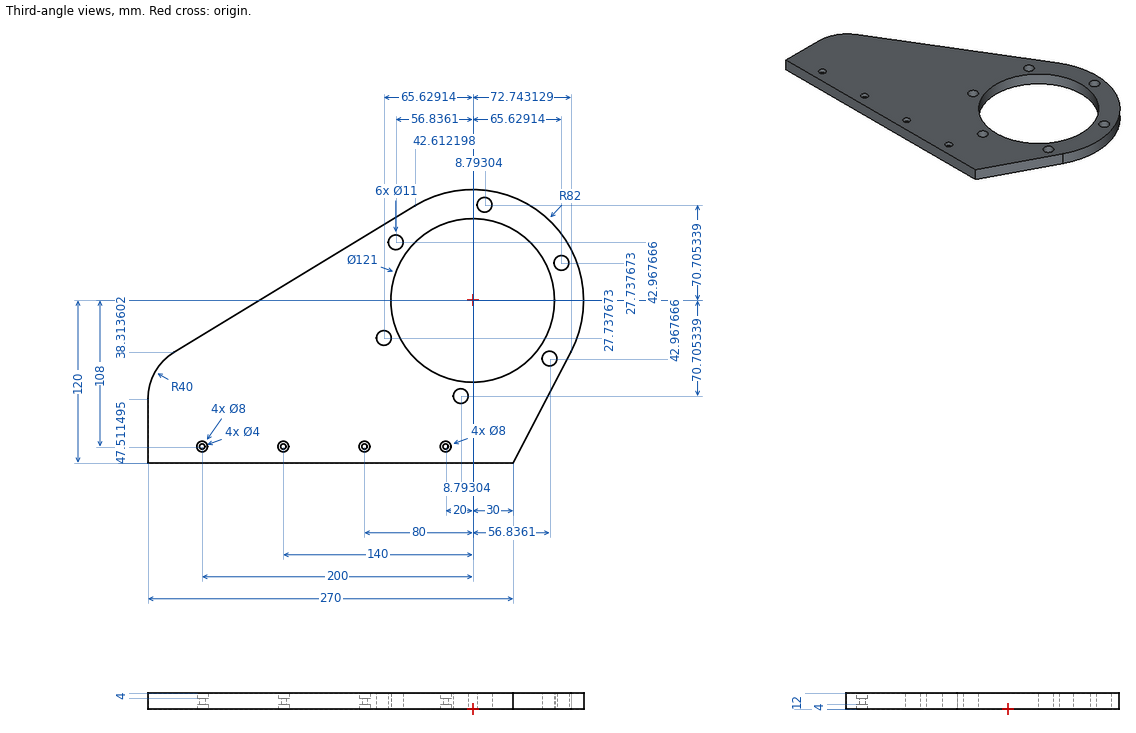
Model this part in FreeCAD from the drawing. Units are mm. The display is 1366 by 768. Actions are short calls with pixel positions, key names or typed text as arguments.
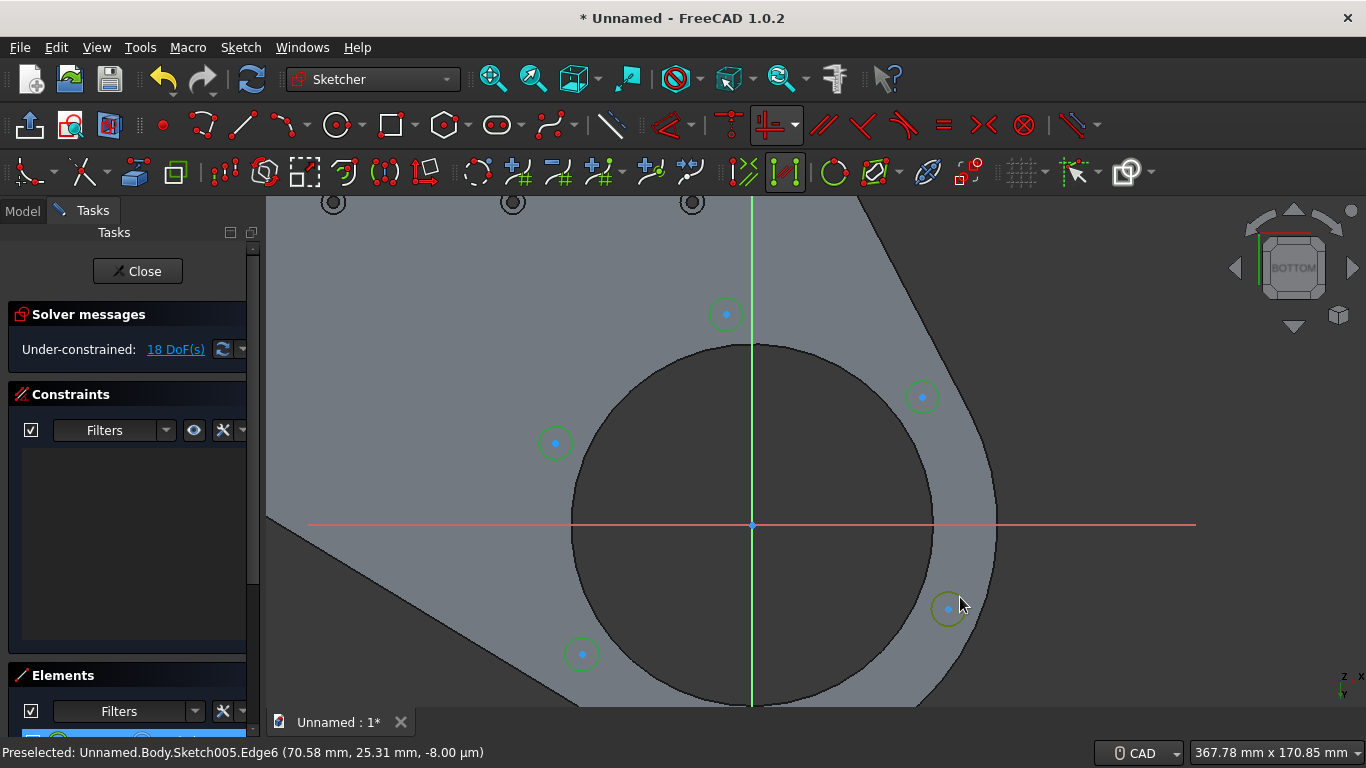
click(944, 126)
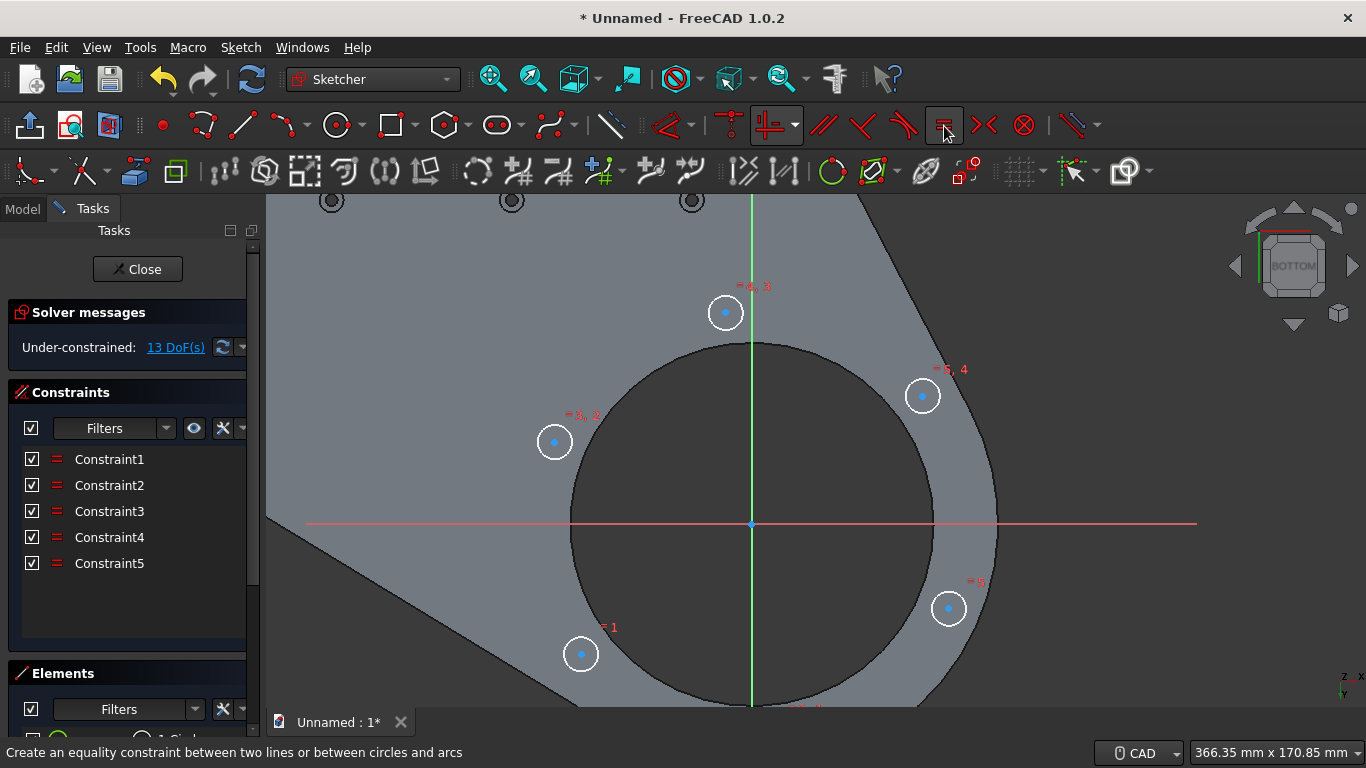
click(666, 126)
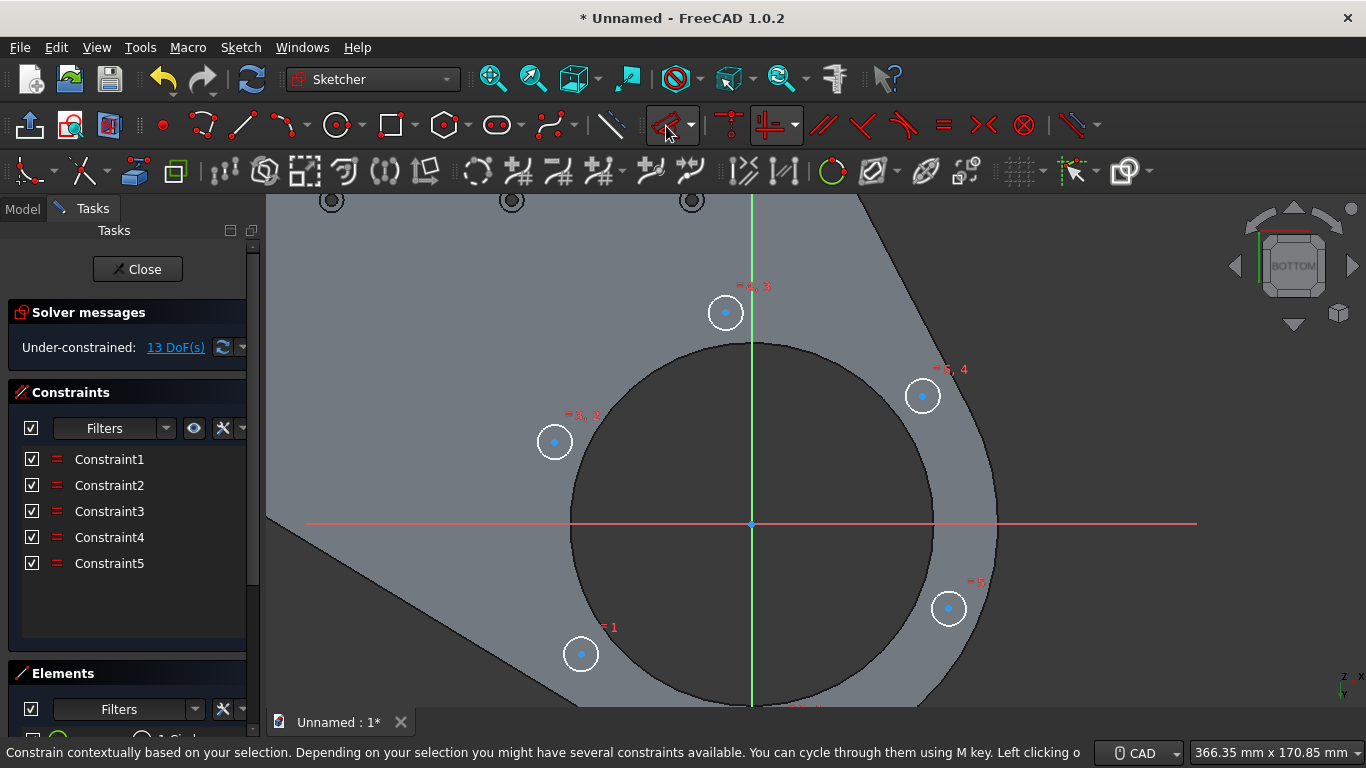
click(593, 642)
click(615, 619)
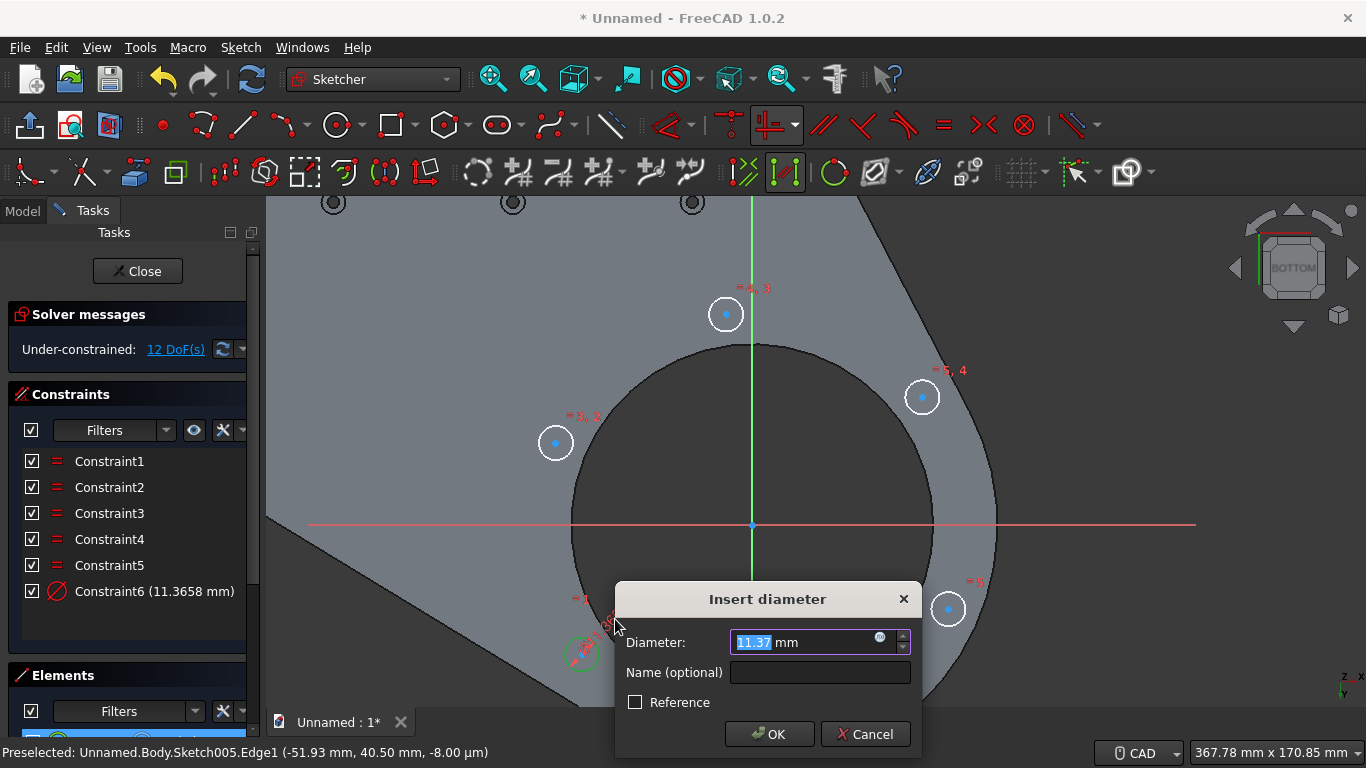
text(11)
key(Return)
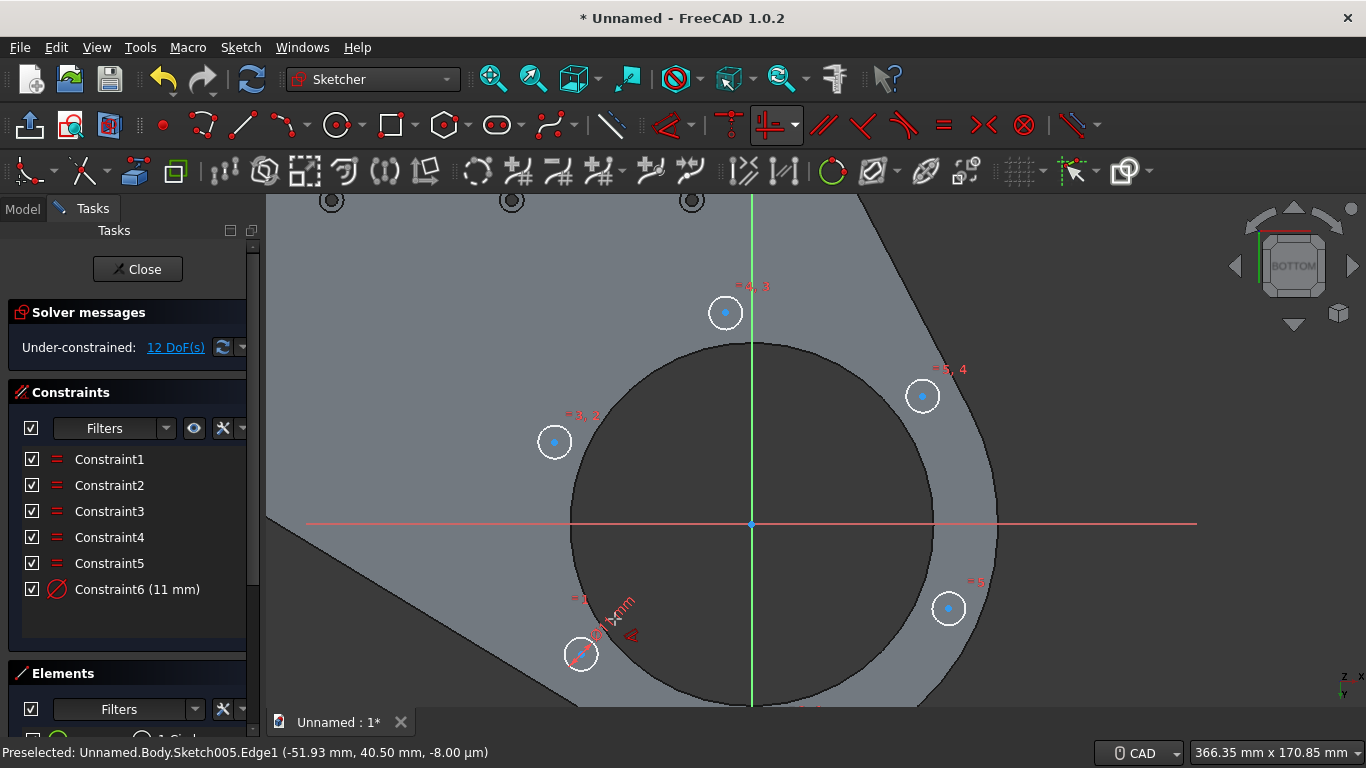
click(581, 654)
click(667, 490)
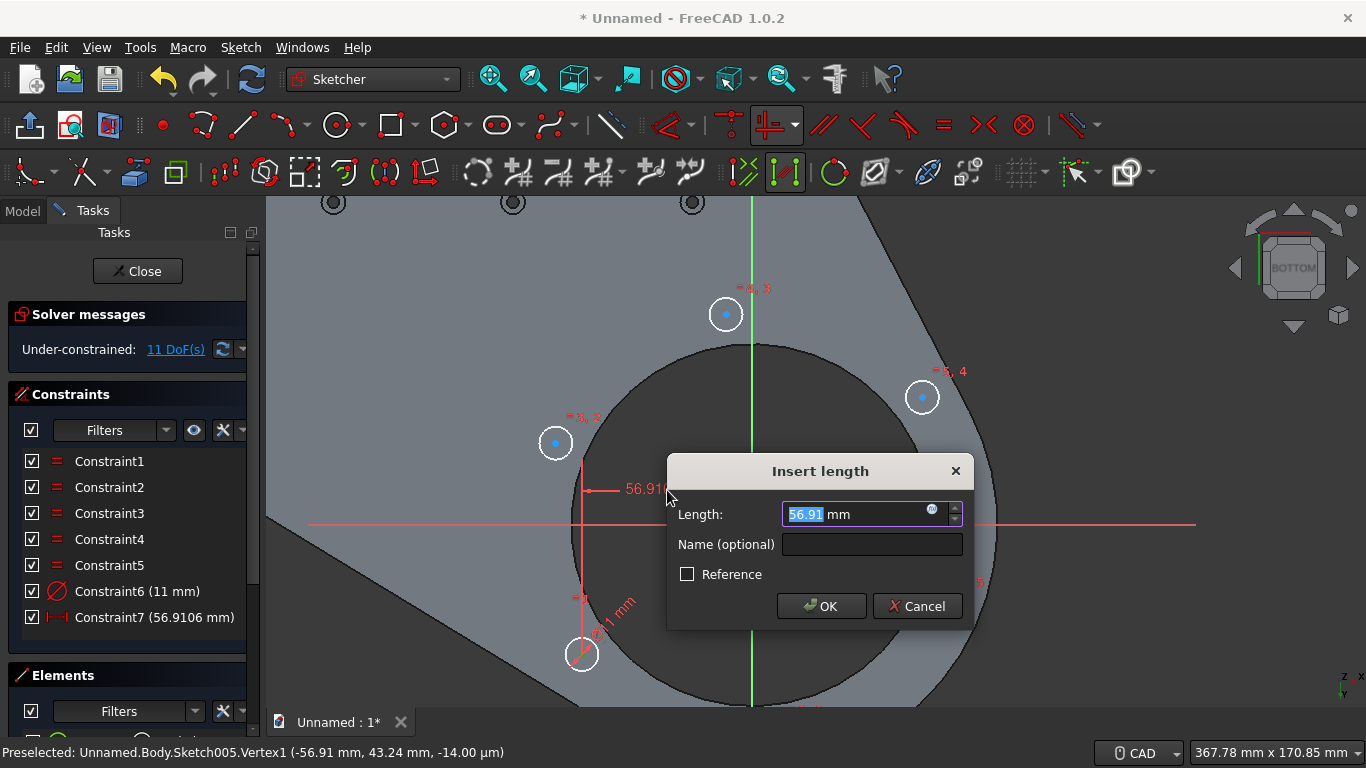
text(56.8361)
key(Return)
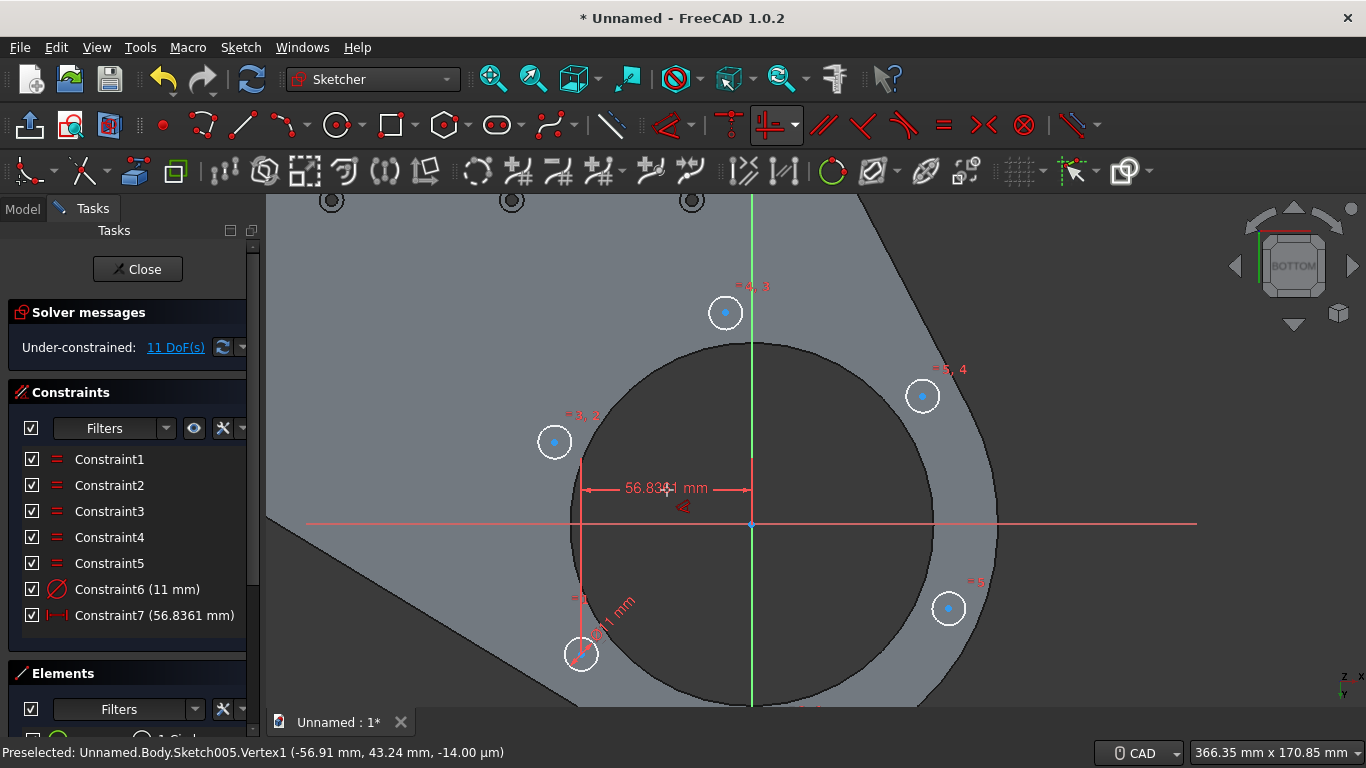
scroll(738, 300, down, 2)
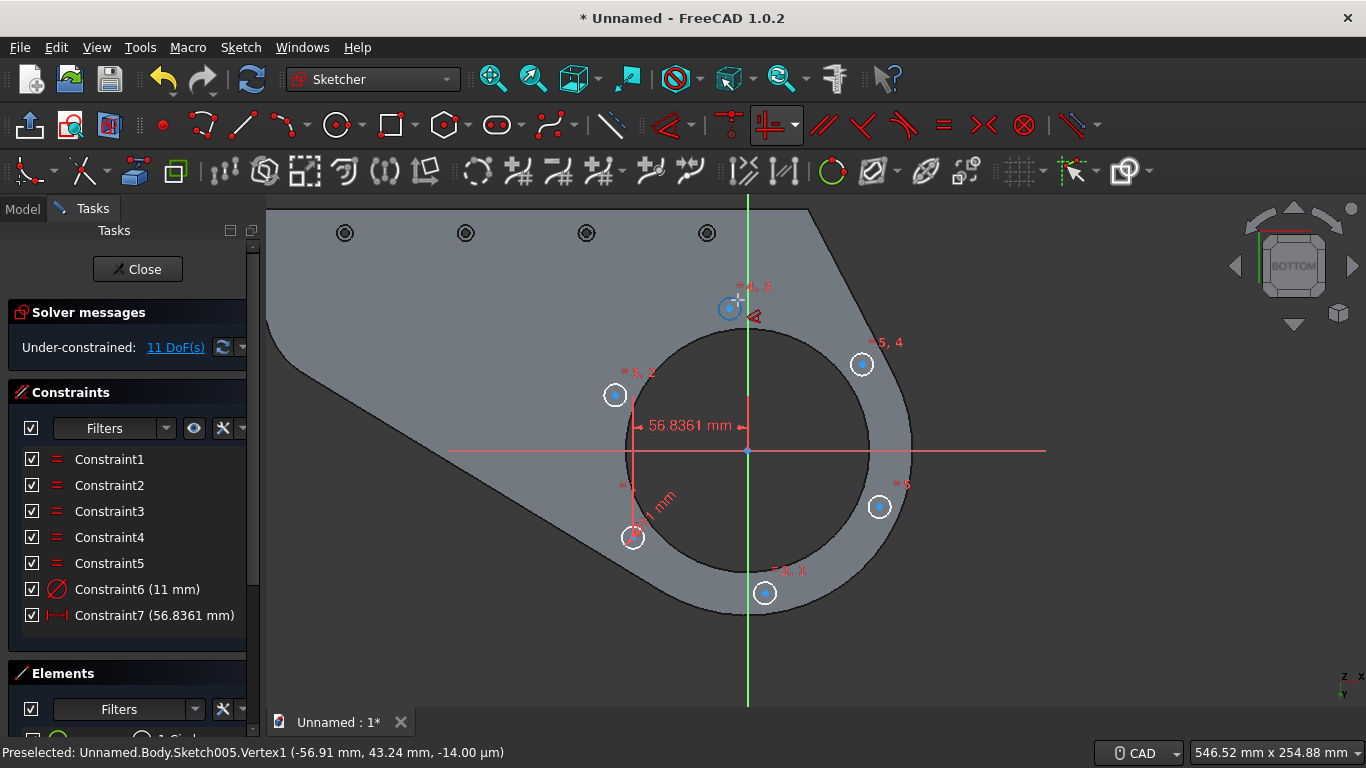
scroll(765, 593, up, 5)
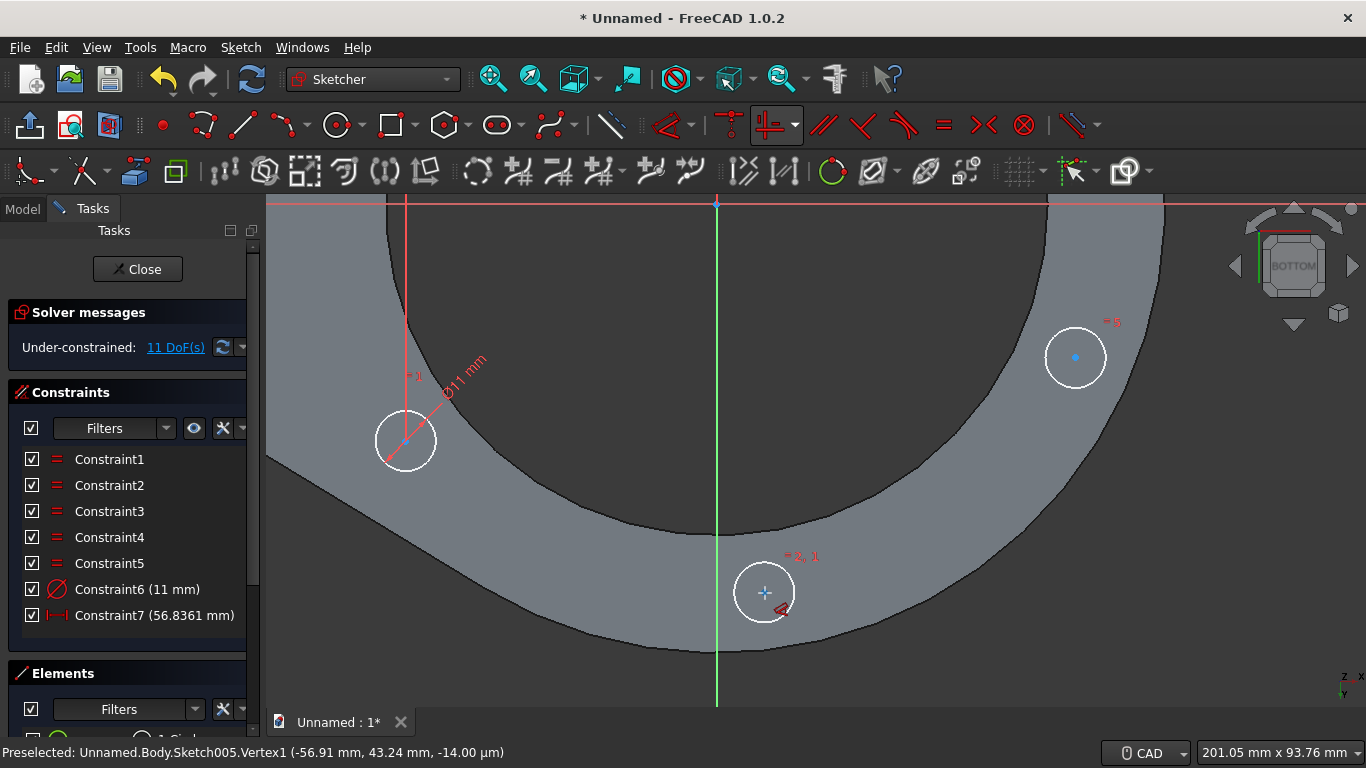
click(764, 592)
click(741, 650)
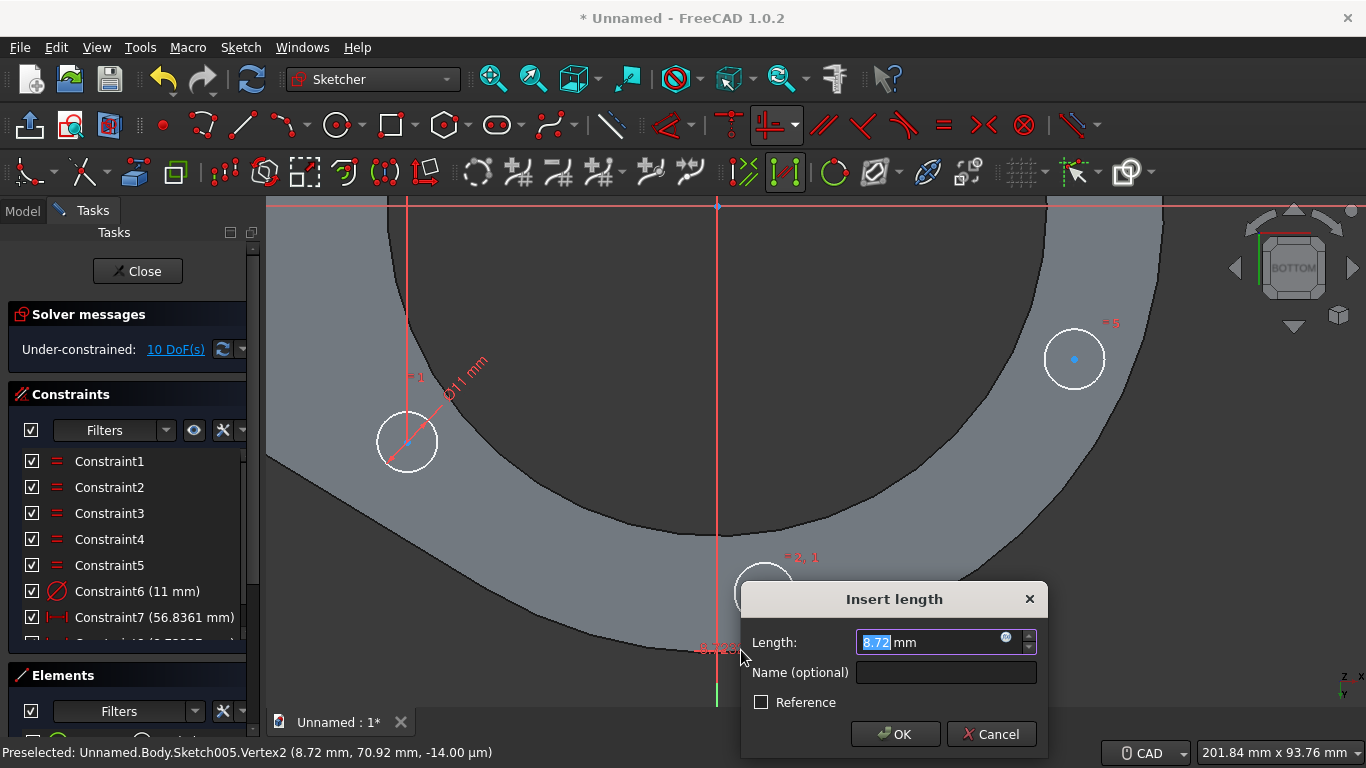
text(8.79304)
key(Return)